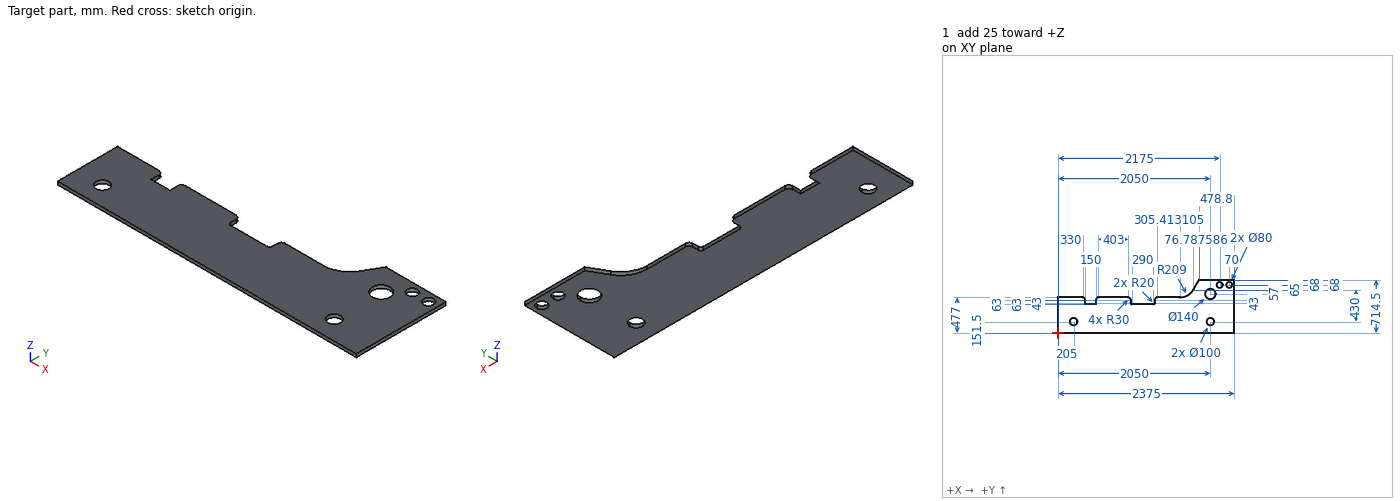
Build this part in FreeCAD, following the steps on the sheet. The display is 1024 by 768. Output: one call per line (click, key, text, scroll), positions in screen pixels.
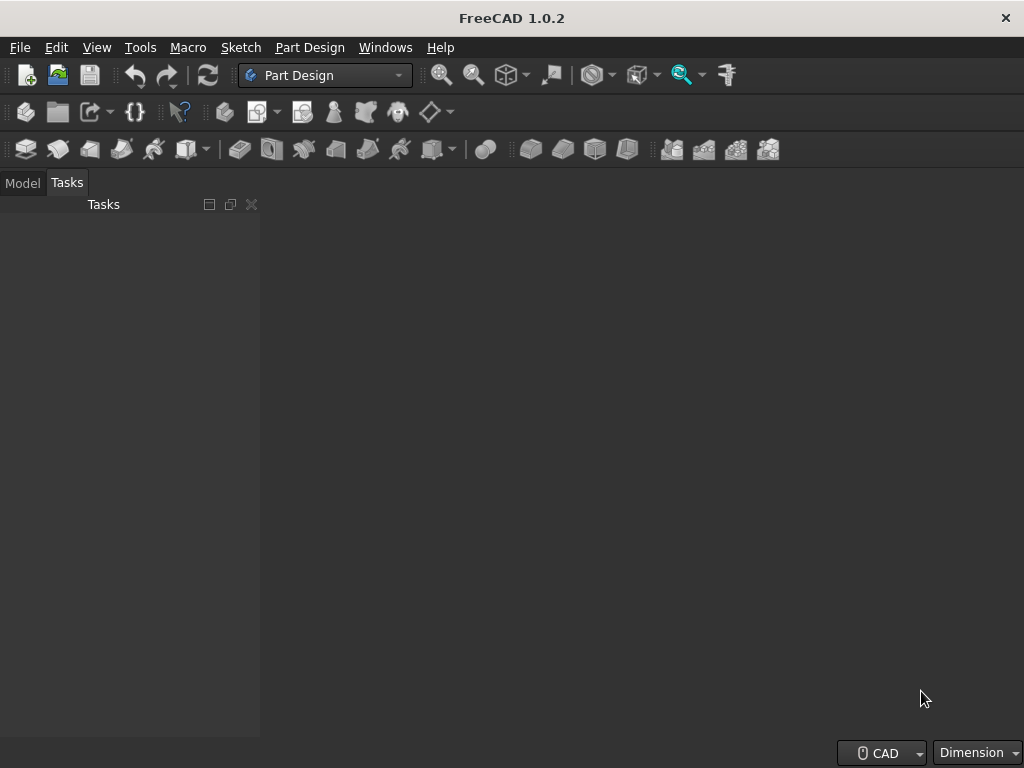
click(26, 76)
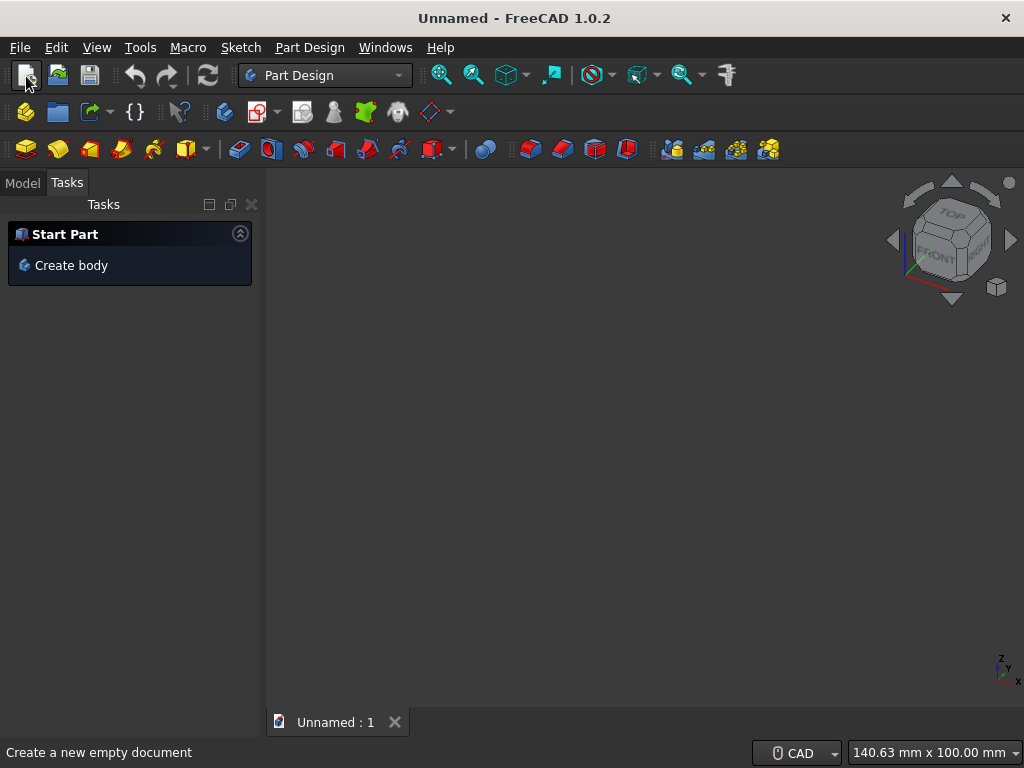
click(258, 112)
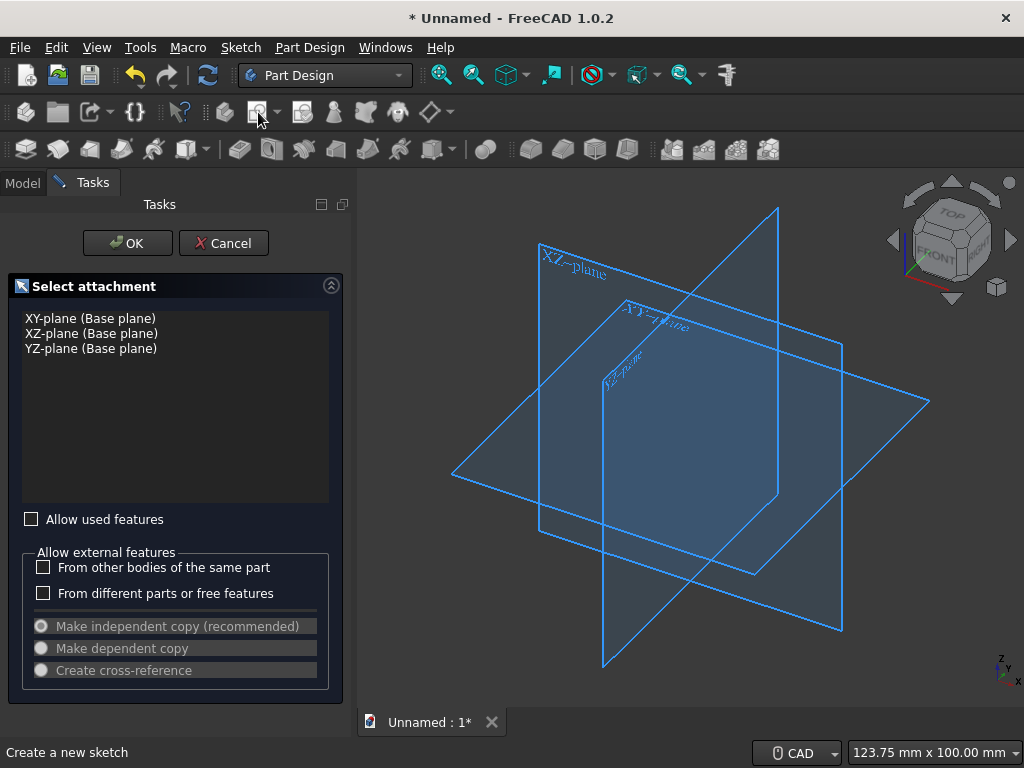
click(82, 318)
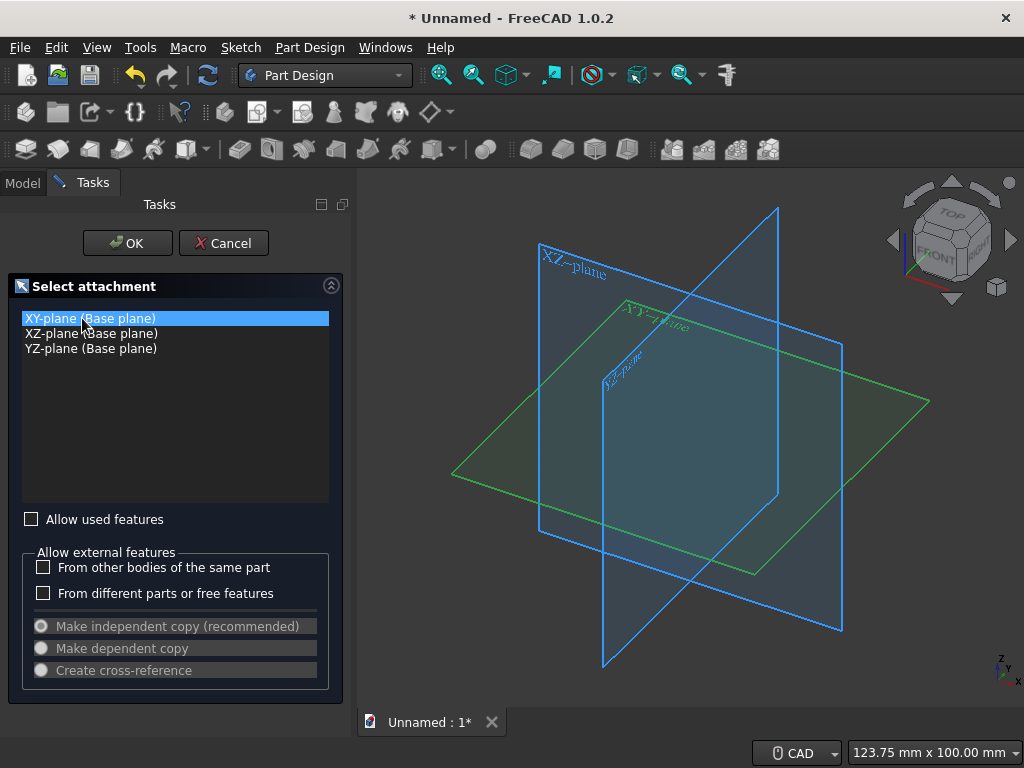
click(128, 243)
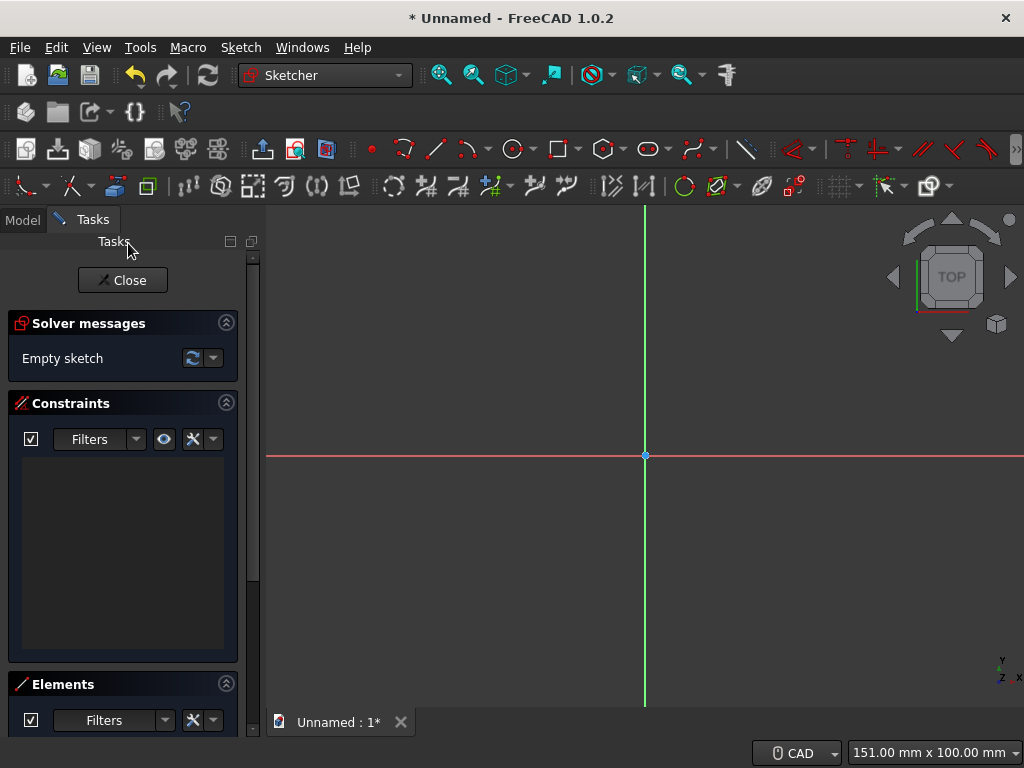
scroll(320, 532, down, 16)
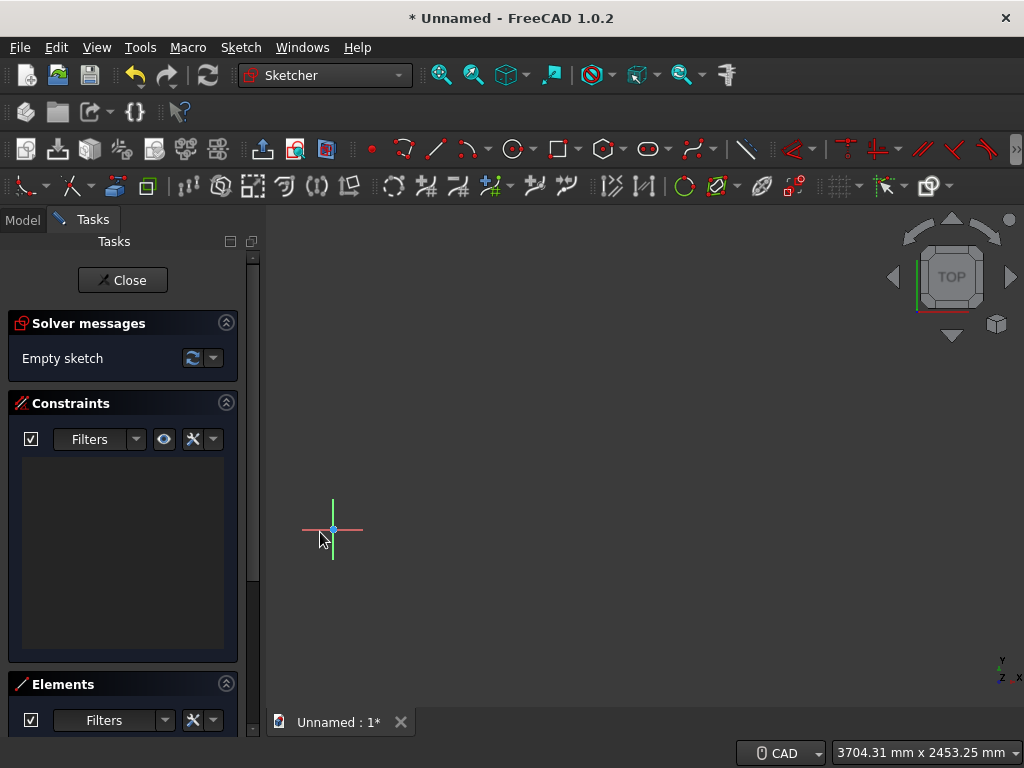
click(436, 150)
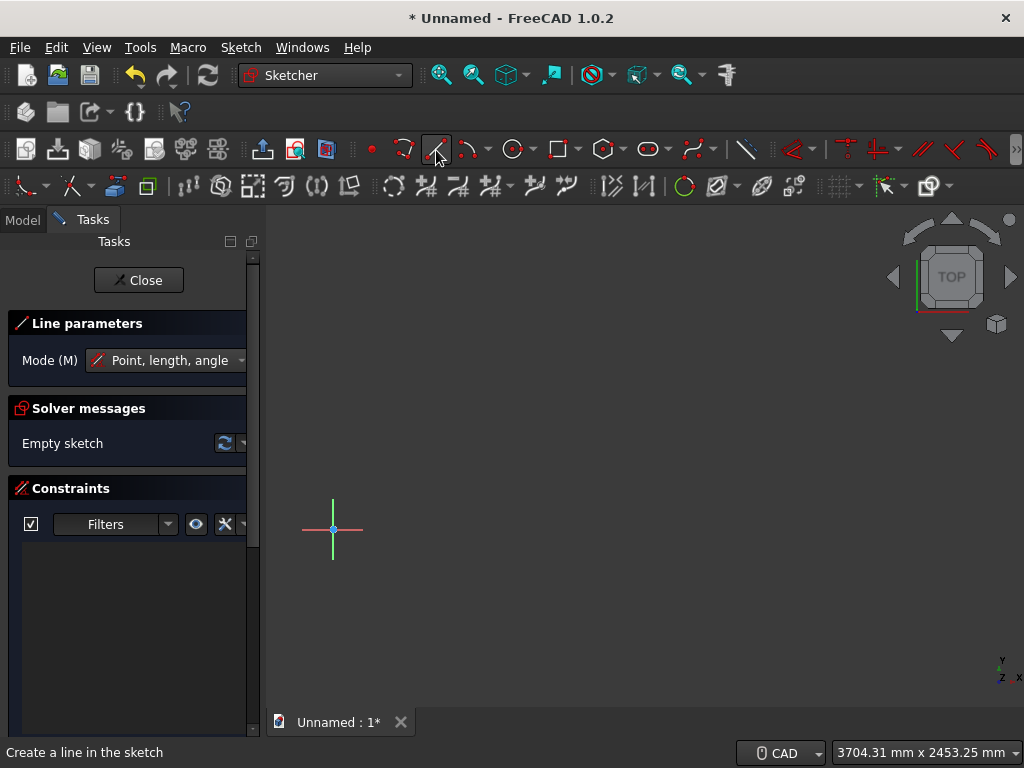
click(669, 432)
click(606, 432)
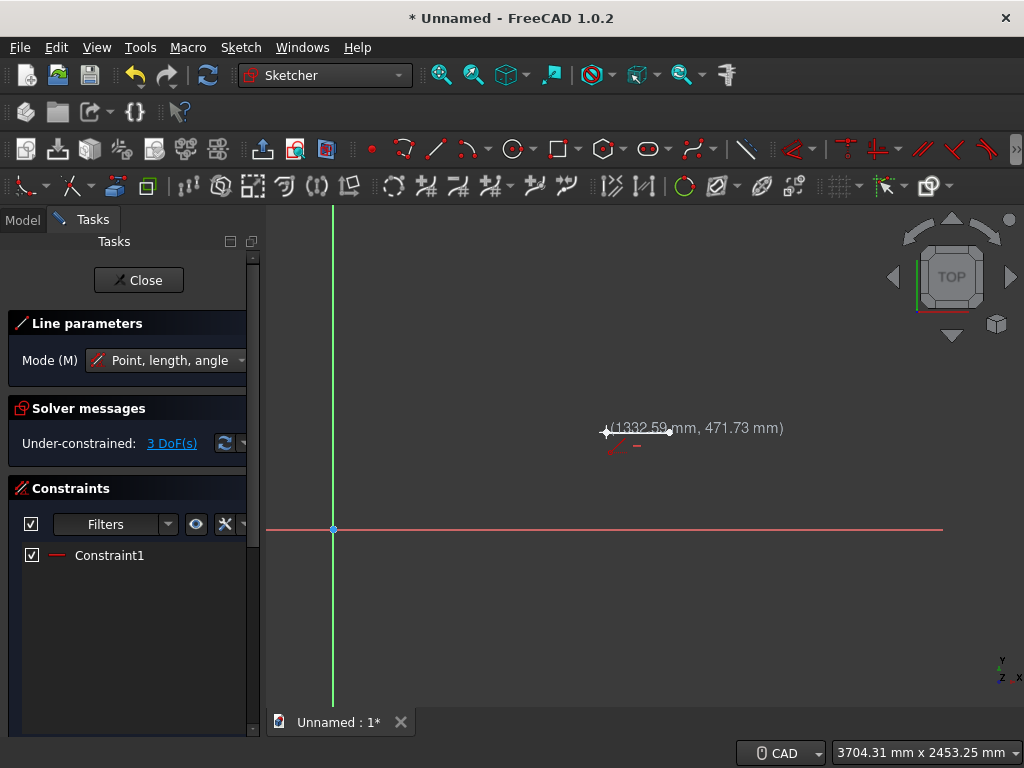
scroll(600, 438, up, 4)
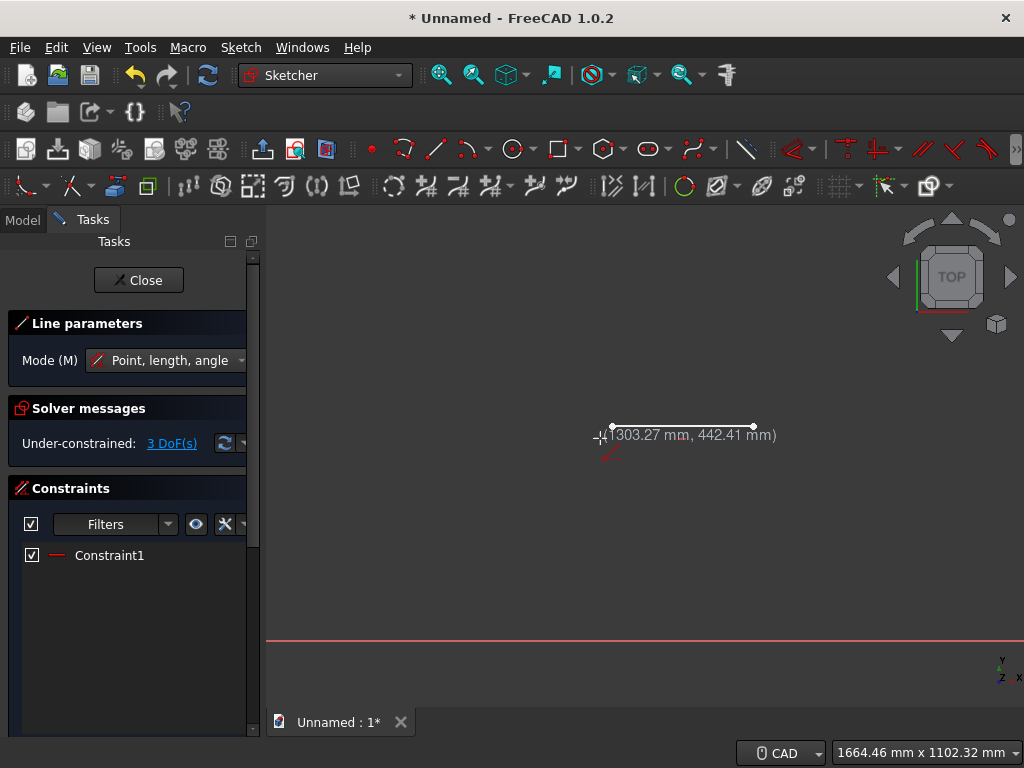
click(599, 438)
click(599, 457)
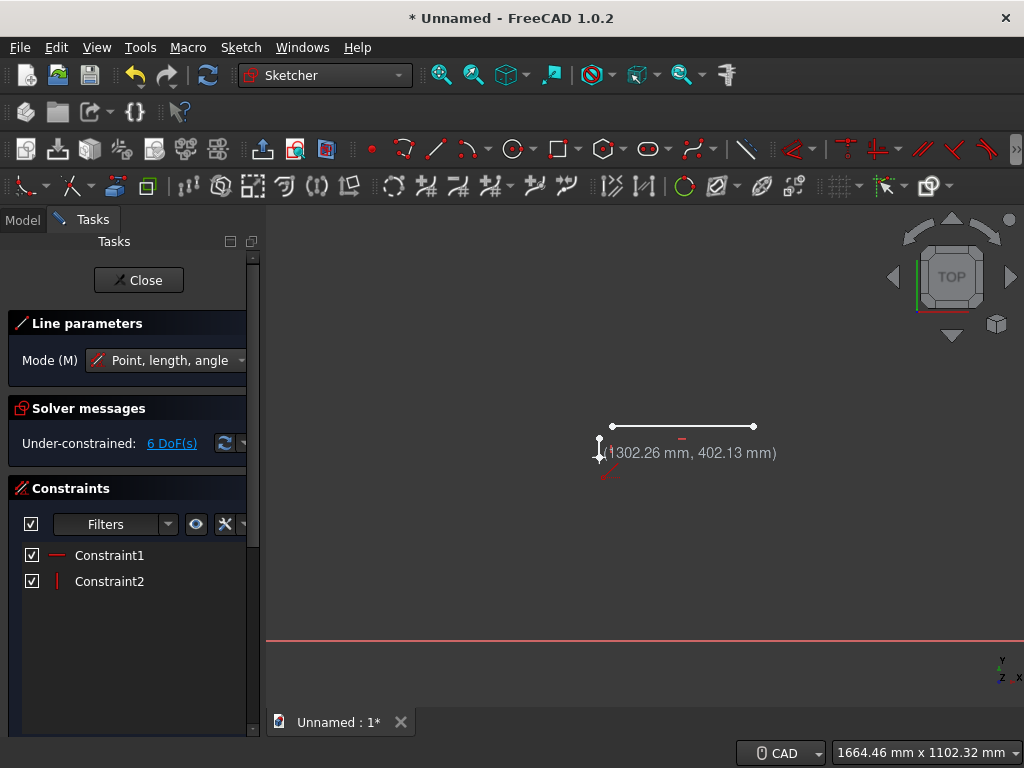
scroll(590, 466, up, 2)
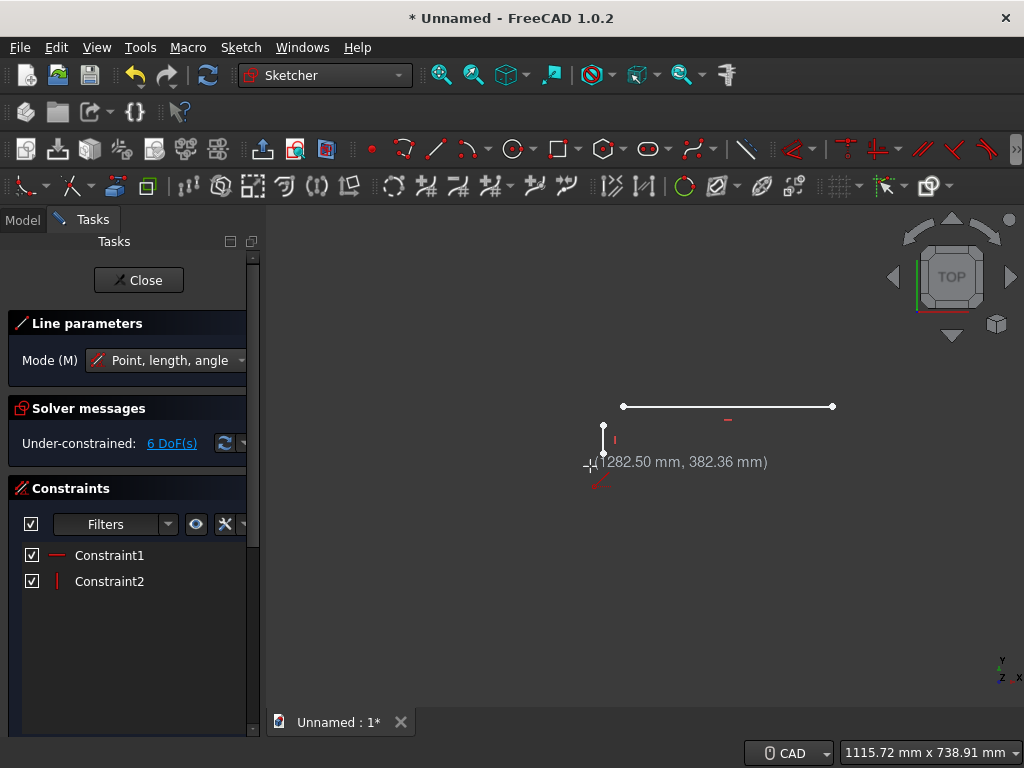
click(590, 466)
click(393, 466)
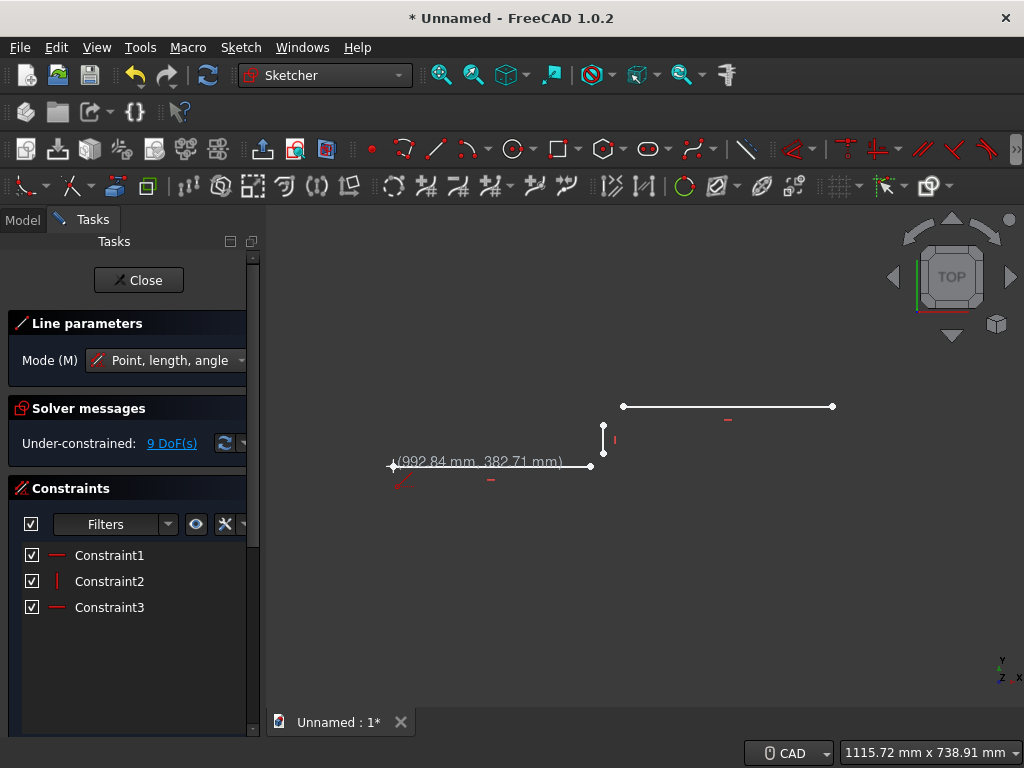
click(380, 453)
click(380, 423)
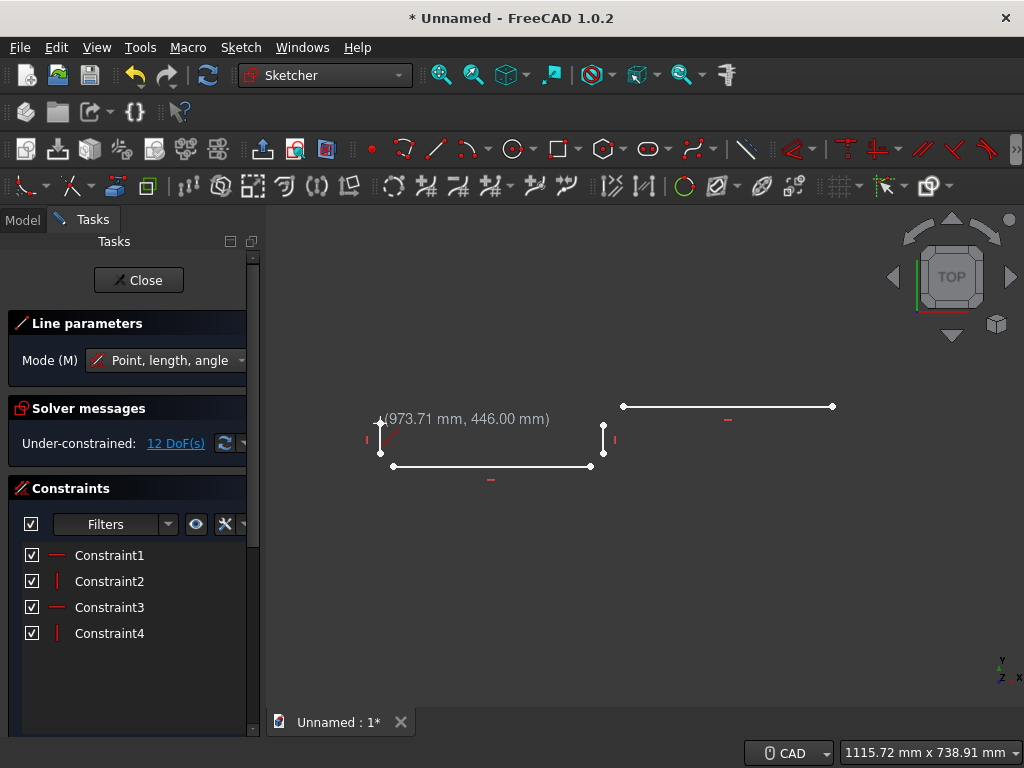
click(359, 403)